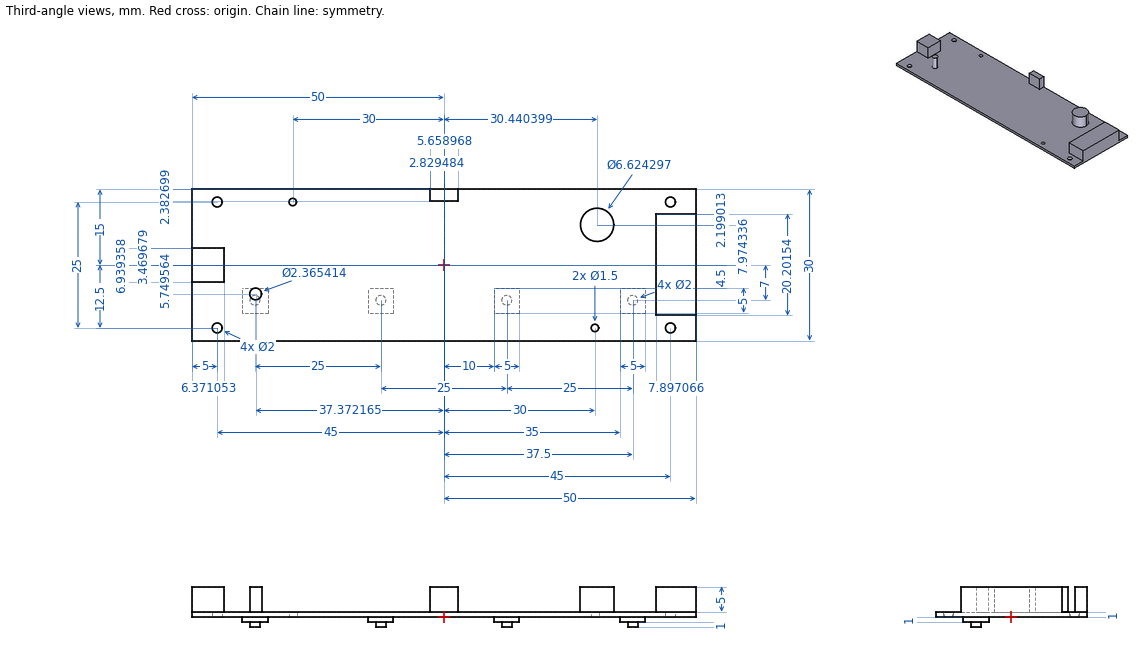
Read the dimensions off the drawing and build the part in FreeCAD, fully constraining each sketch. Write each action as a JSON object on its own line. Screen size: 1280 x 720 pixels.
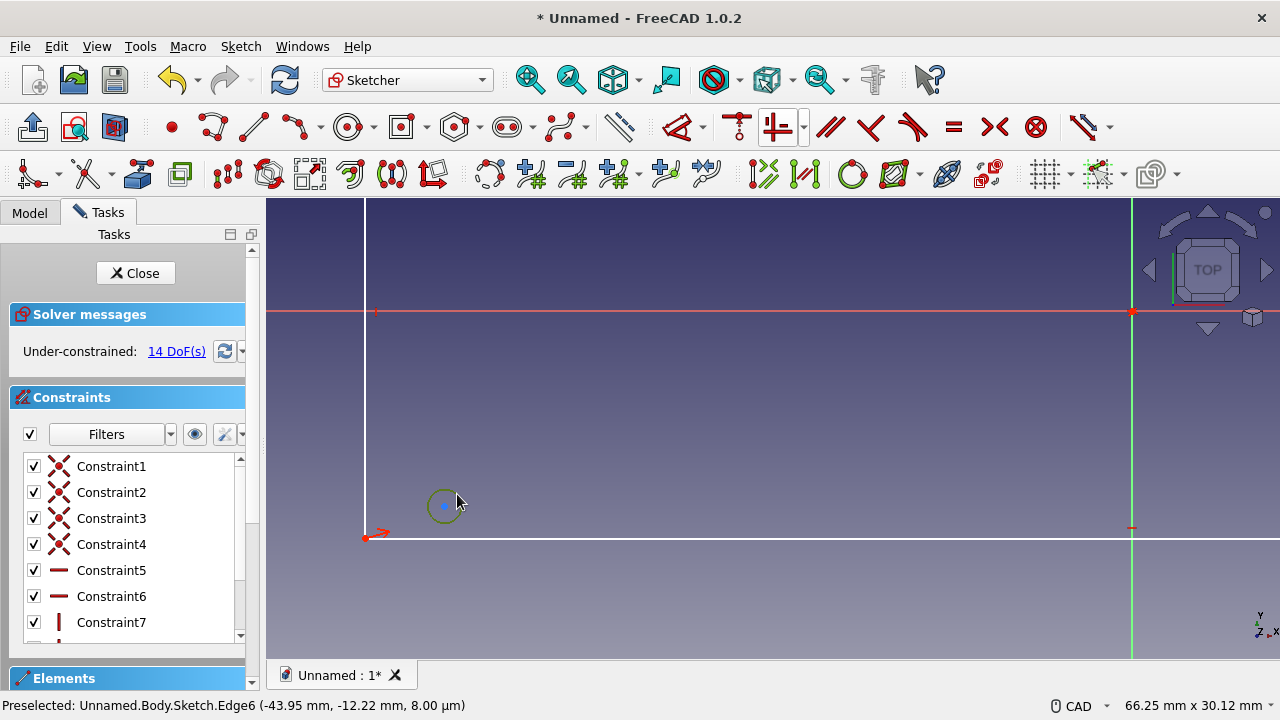
{"action": "scroll", "coordinate": [456, 497], "scroll_direction": "down", "scroll_amount": 5}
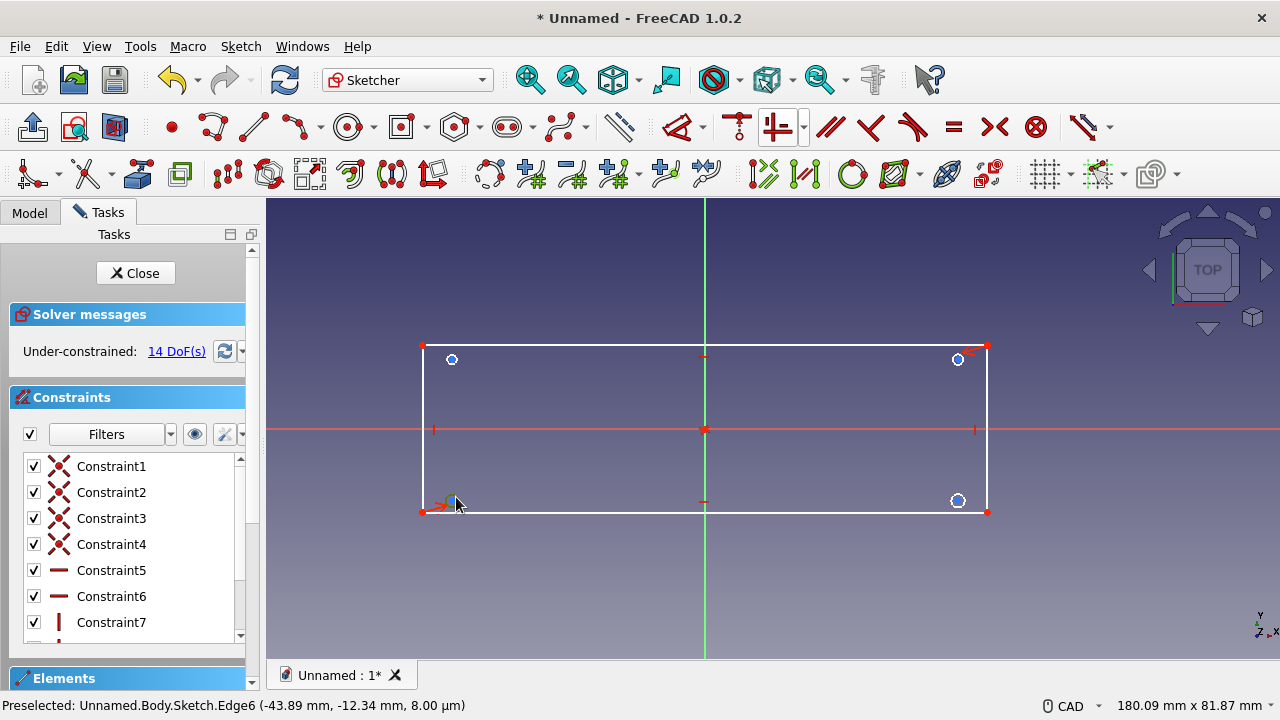
{"action": "scroll", "coordinate": [963, 496], "scroll_direction": "up", "scroll_amount": 4}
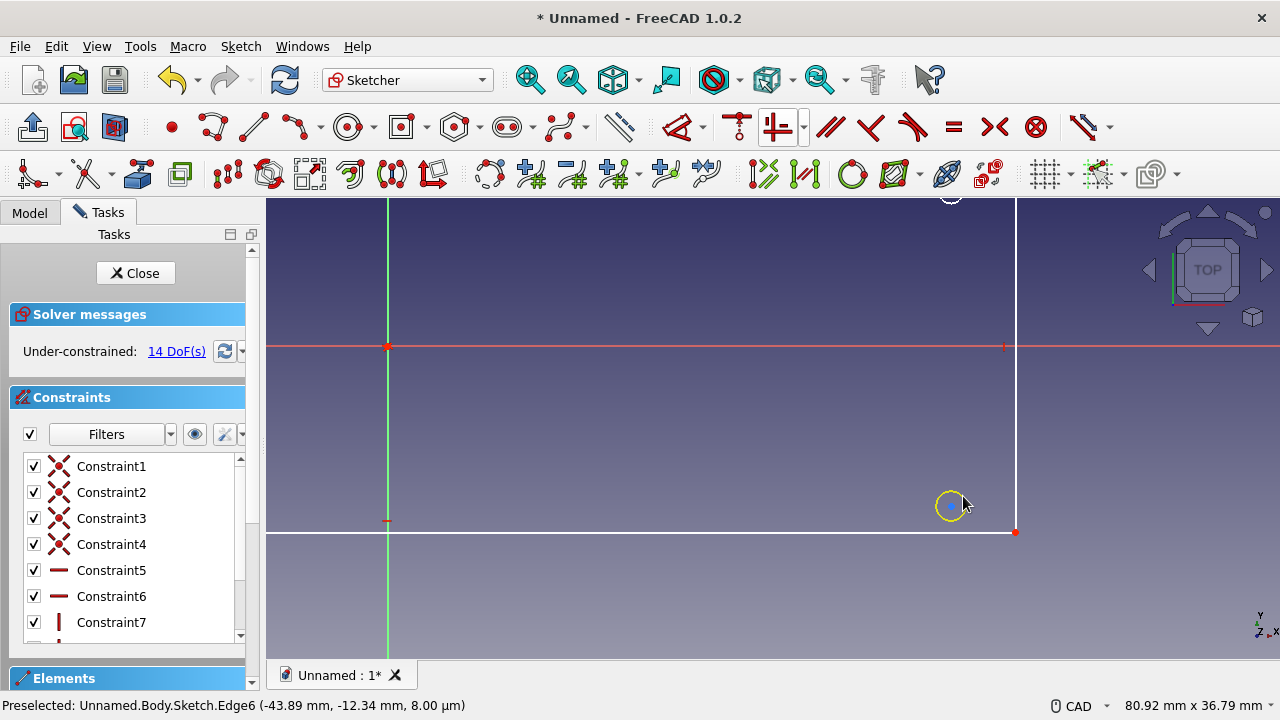
{"action": "left_click", "coordinate": [961, 496]}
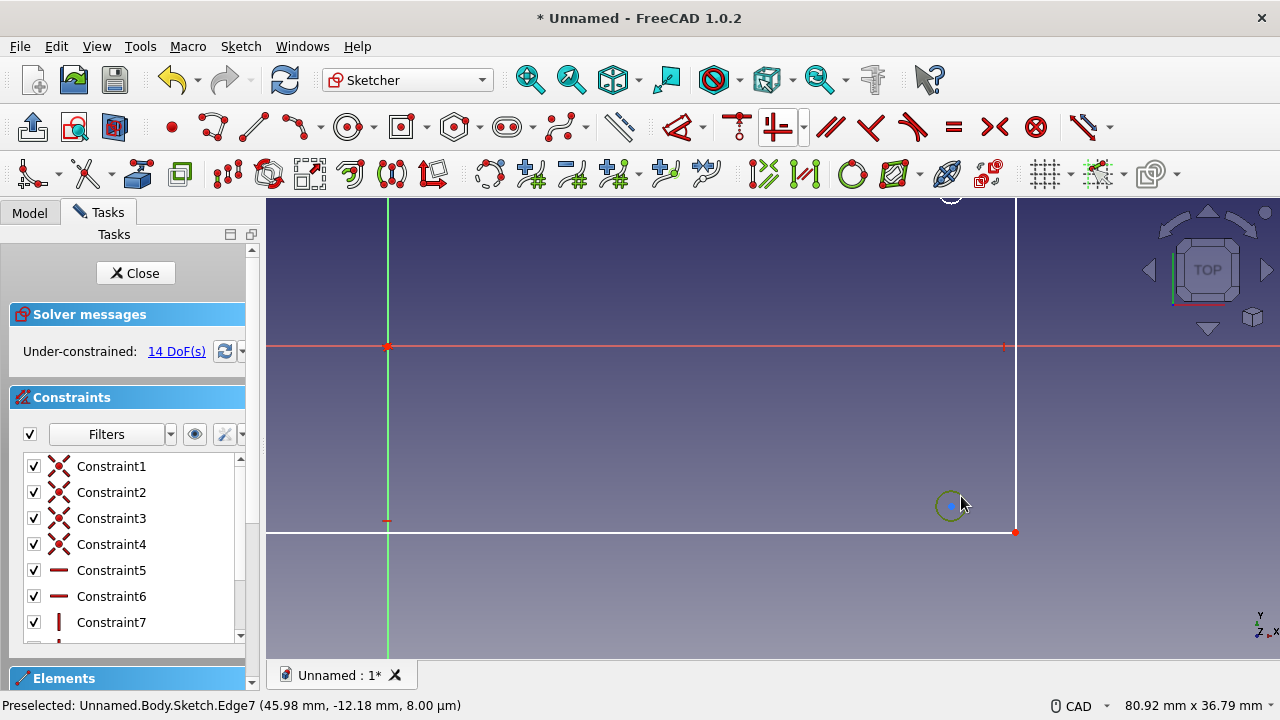
{"action": "scroll", "coordinate": [963, 496], "scroll_direction": "down", "scroll_amount": 4}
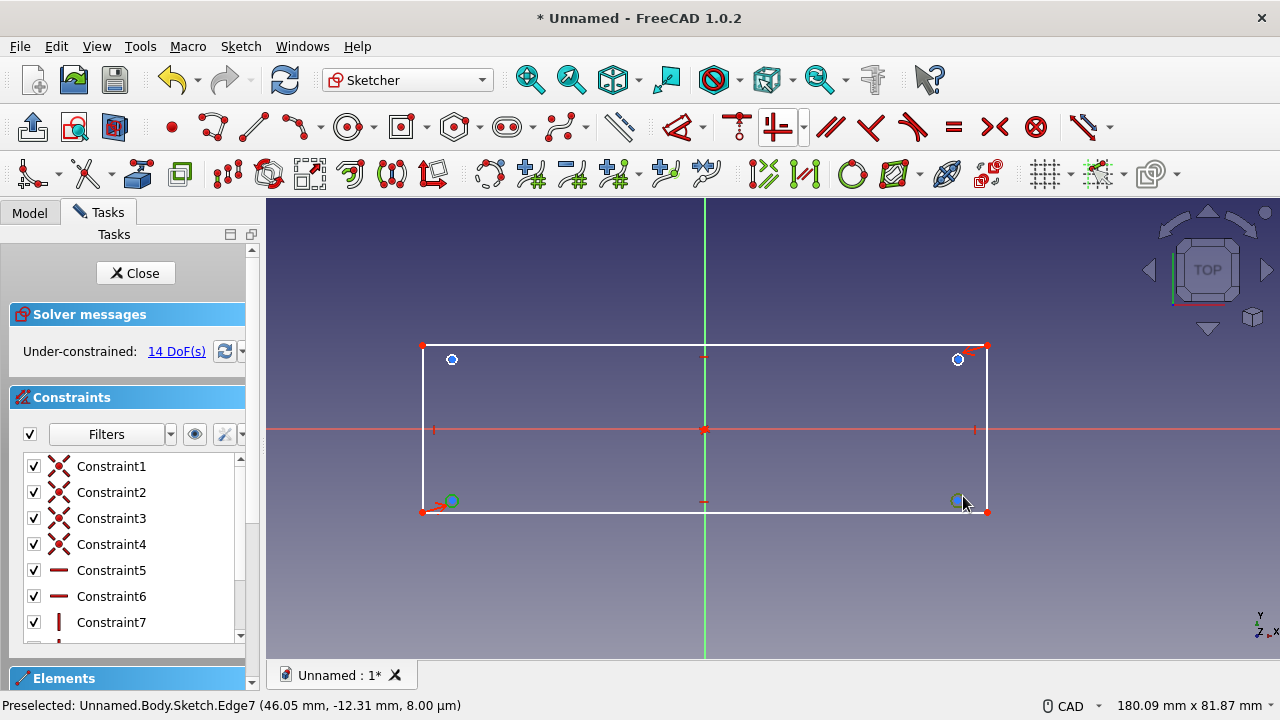
{"action": "scroll", "coordinate": [455, 356], "scroll_direction": "up", "scroll_amount": 6}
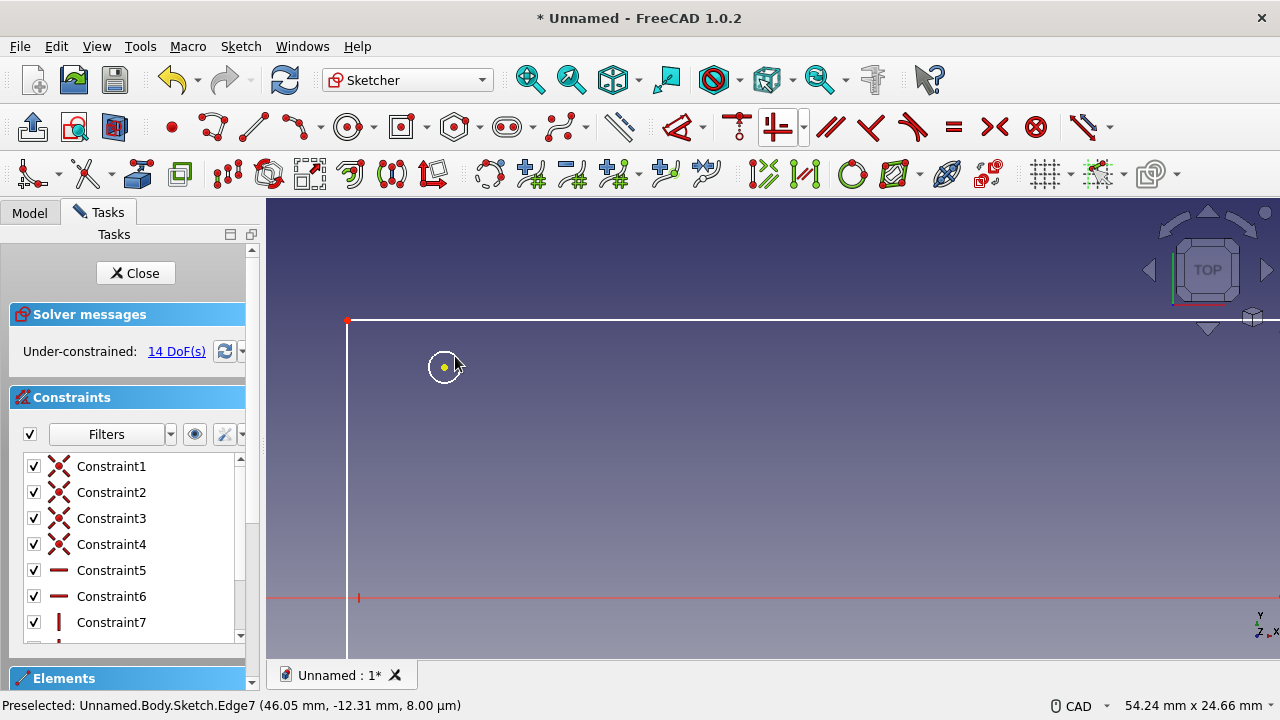
{"action": "left_click", "coordinate": [456, 356]}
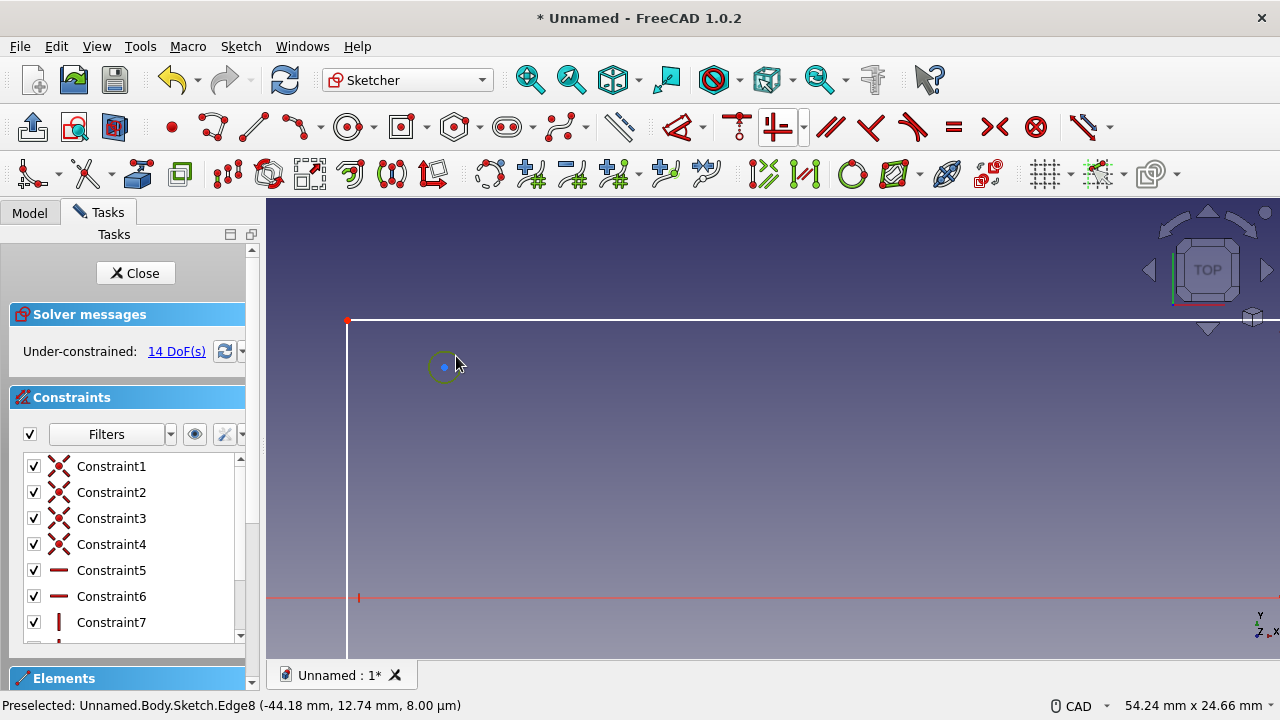
{"action": "scroll", "coordinate": [455, 355], "scroll_direction": "down", "scroll_amount": 6}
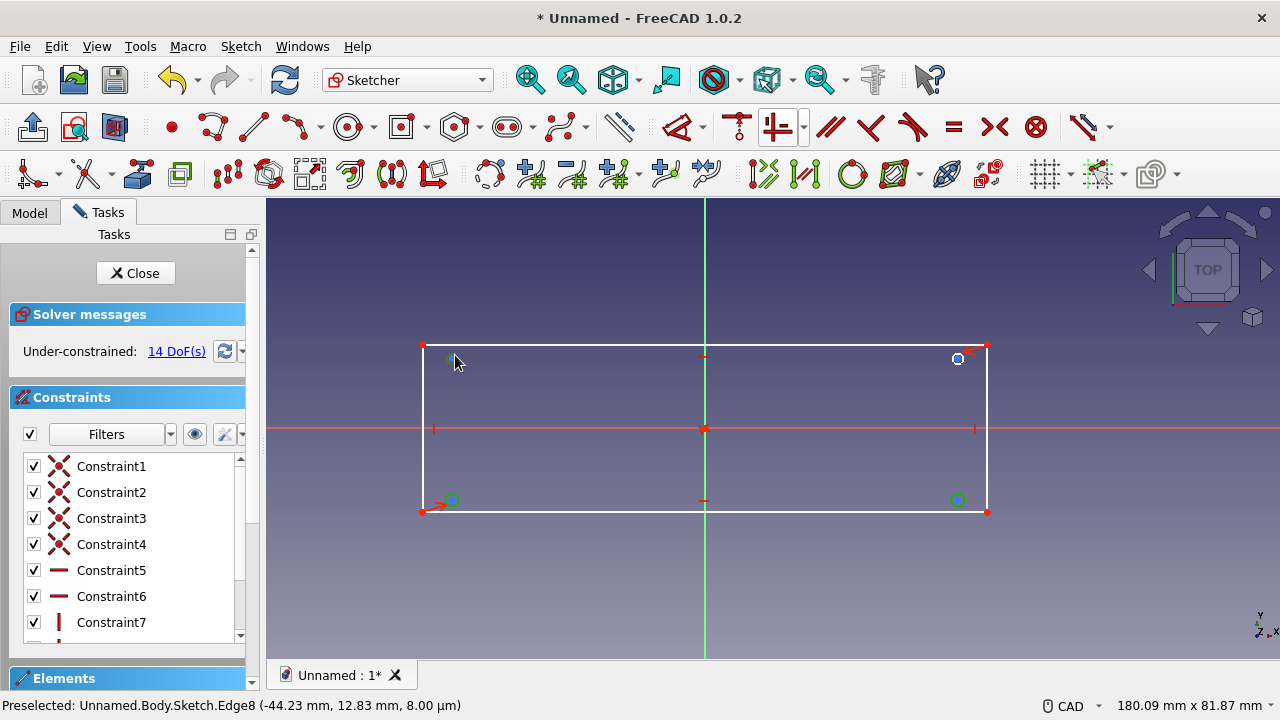
{"action": "scroll", "coordinate": [962, 355], "scroll_direction": "up", "scroll_amount": 5}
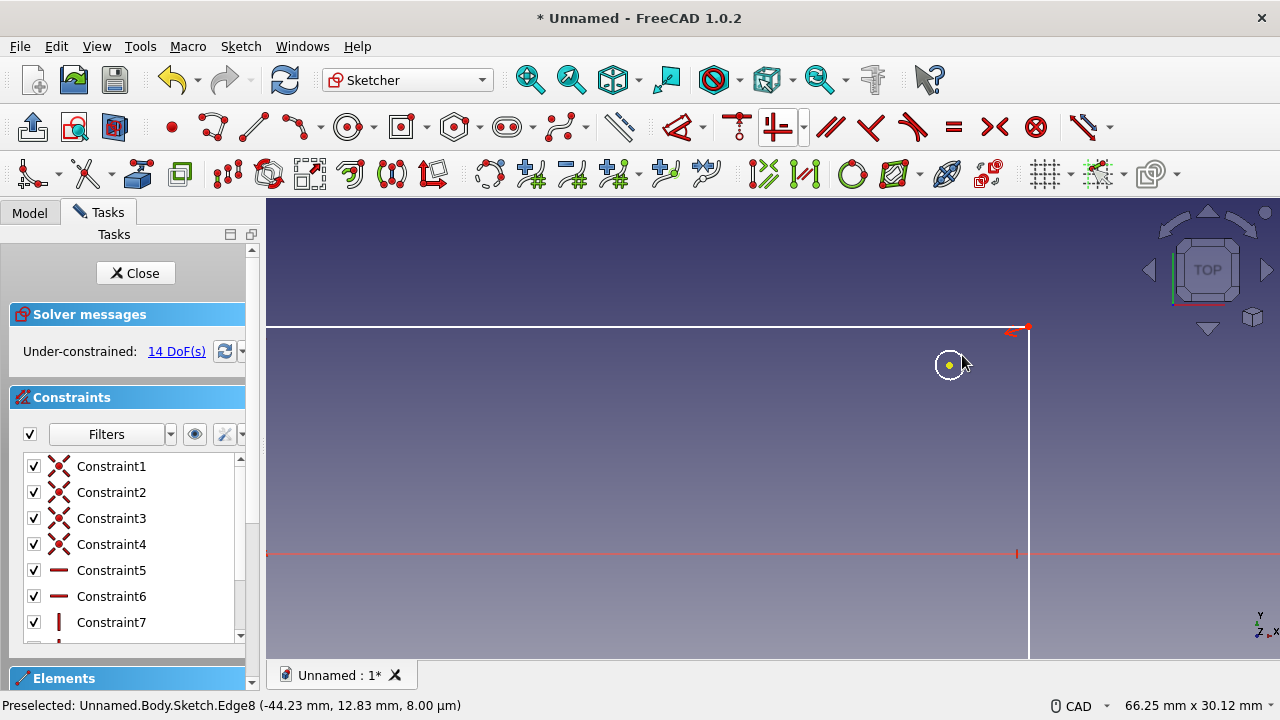
{"action": "left_click", "coordinate": [960, 355]}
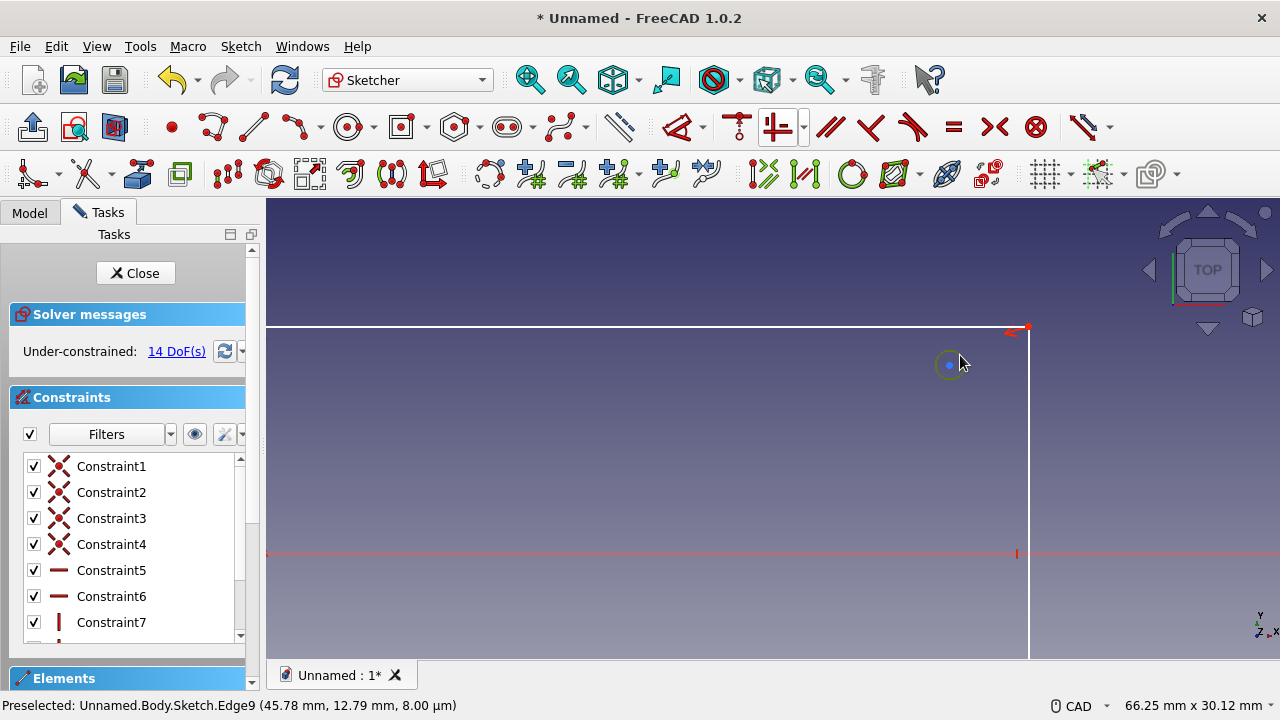
{"action": "left_click", "coordinate": [954, 128]}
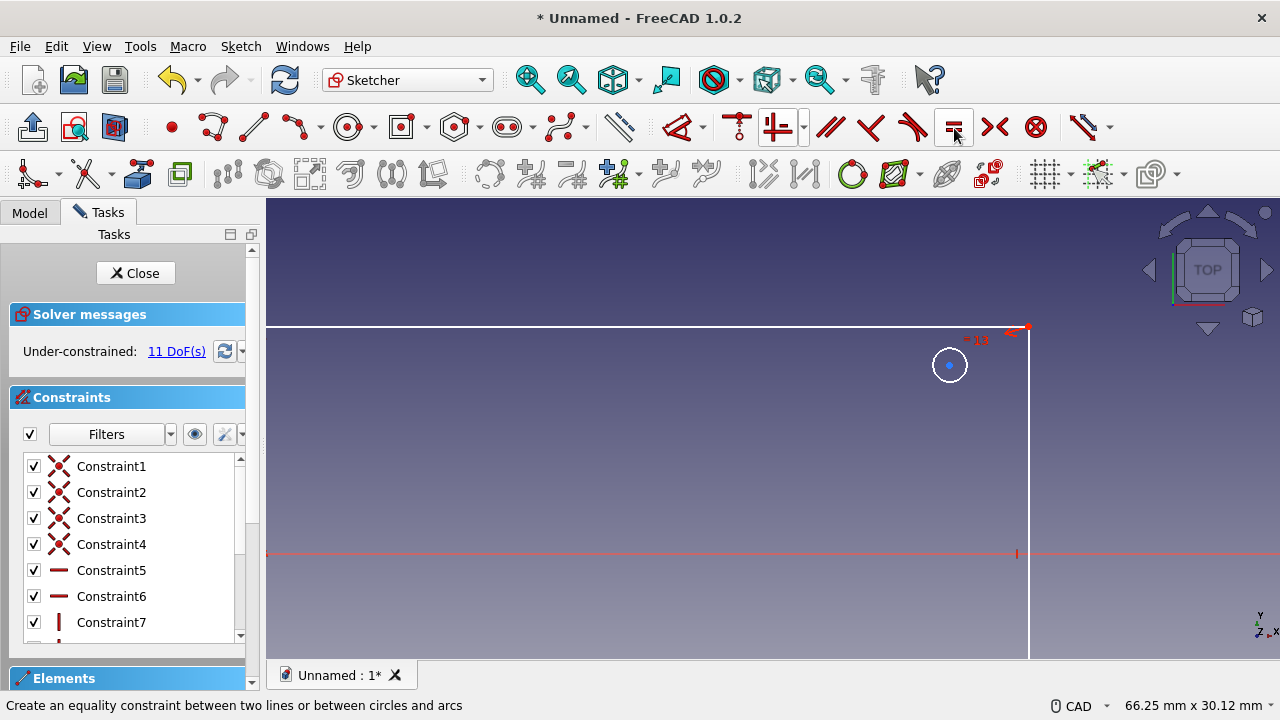
{"action": "scroll", "coordinate": [962, 356], "scroll_direction": "down", "scroll_amount": 5}